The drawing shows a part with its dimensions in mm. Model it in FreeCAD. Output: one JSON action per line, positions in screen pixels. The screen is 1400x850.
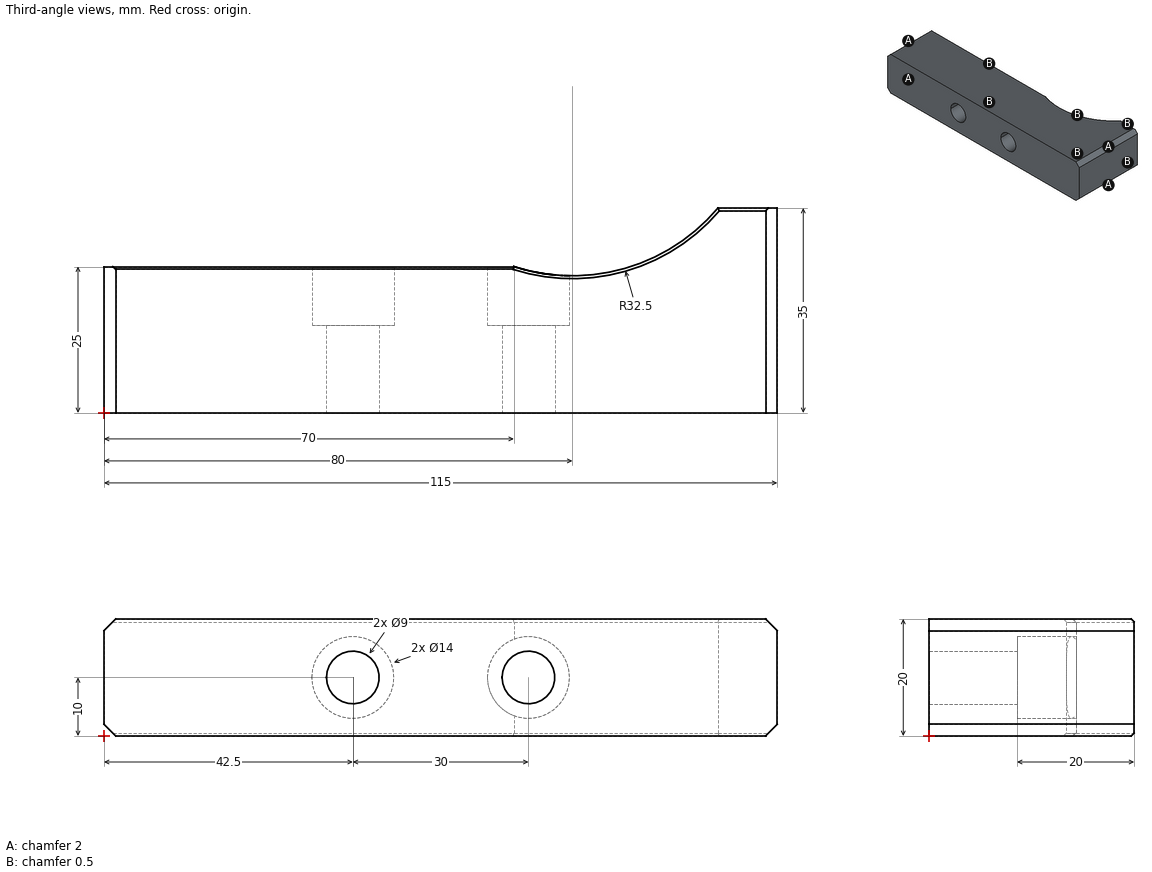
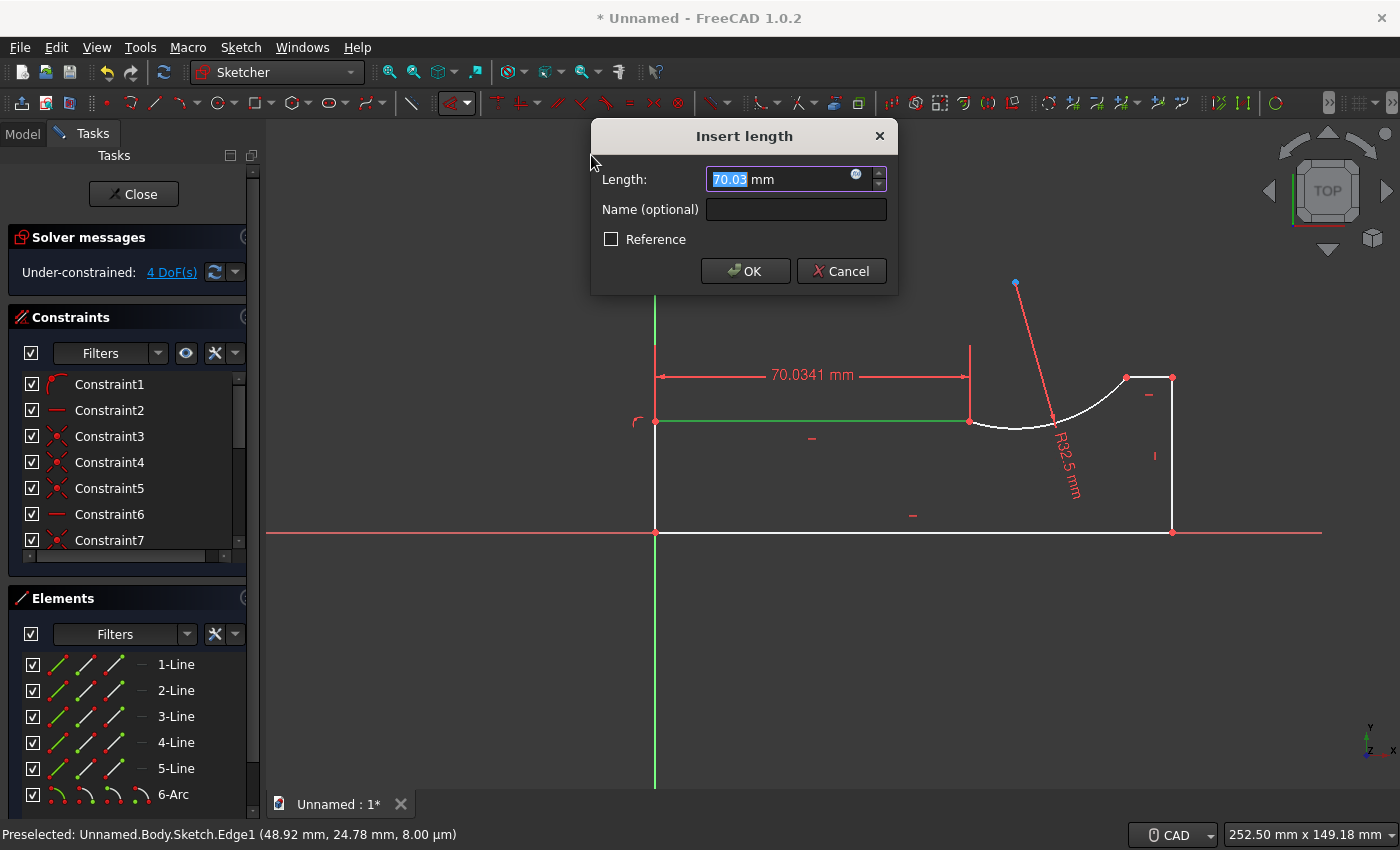
{"action": "type", "text": "70"}
{"action": "key", "text": "Return"}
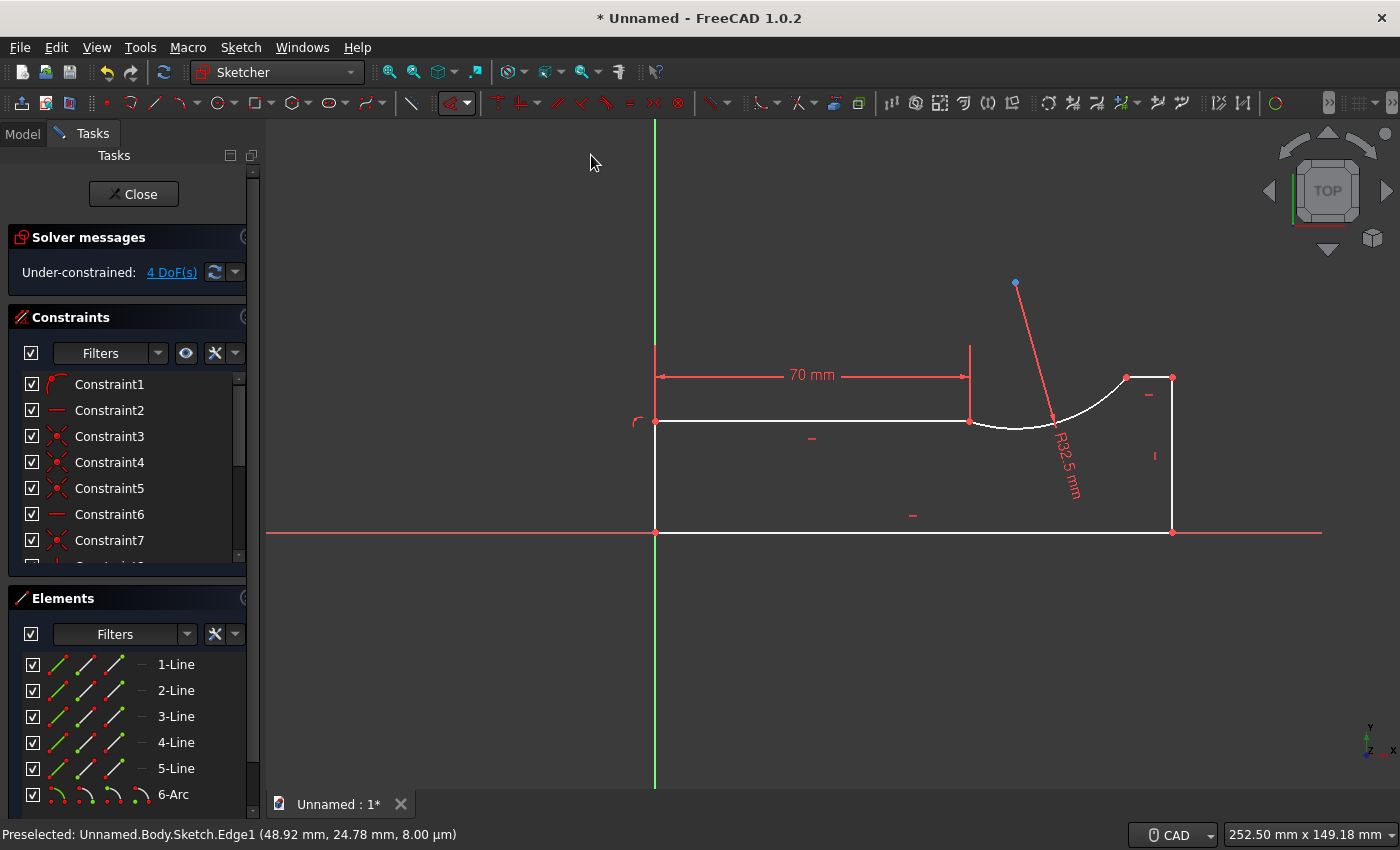
{"action": "left_click", "coordinate": [655, 455]}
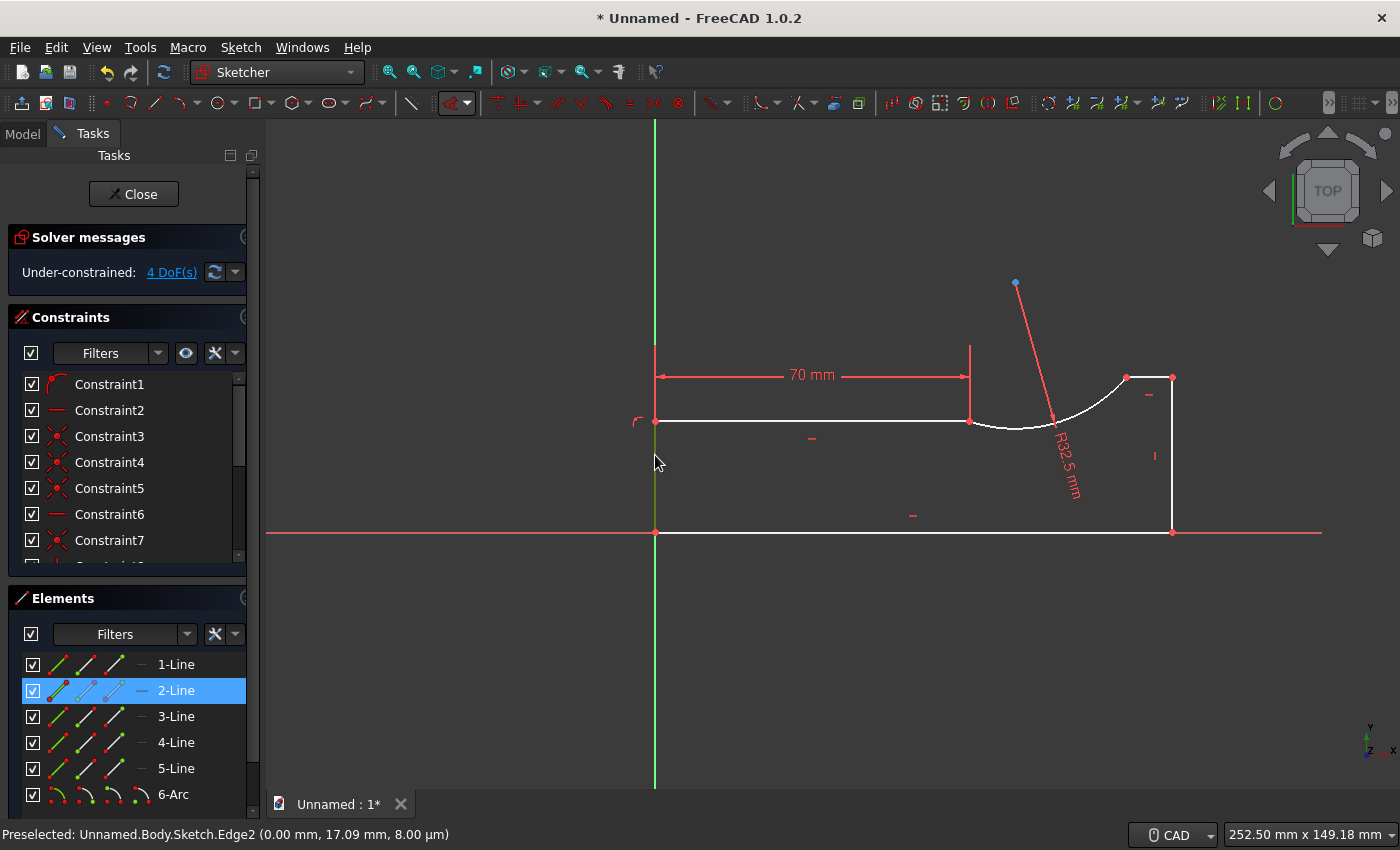
{"action": "key", "text": "i"}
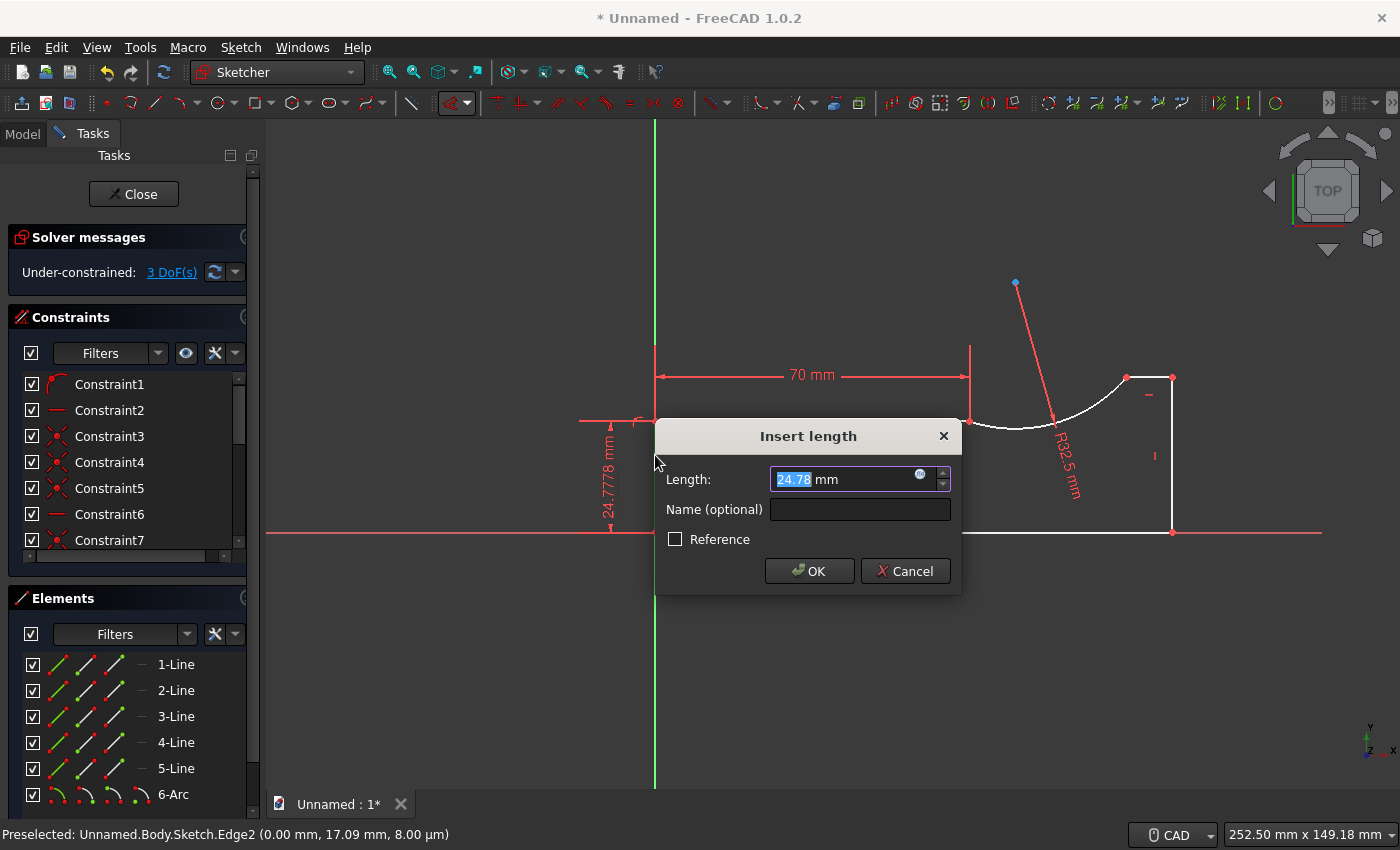
{"action": "type", "text": "25"}
{"action": "key", "text": "Return"}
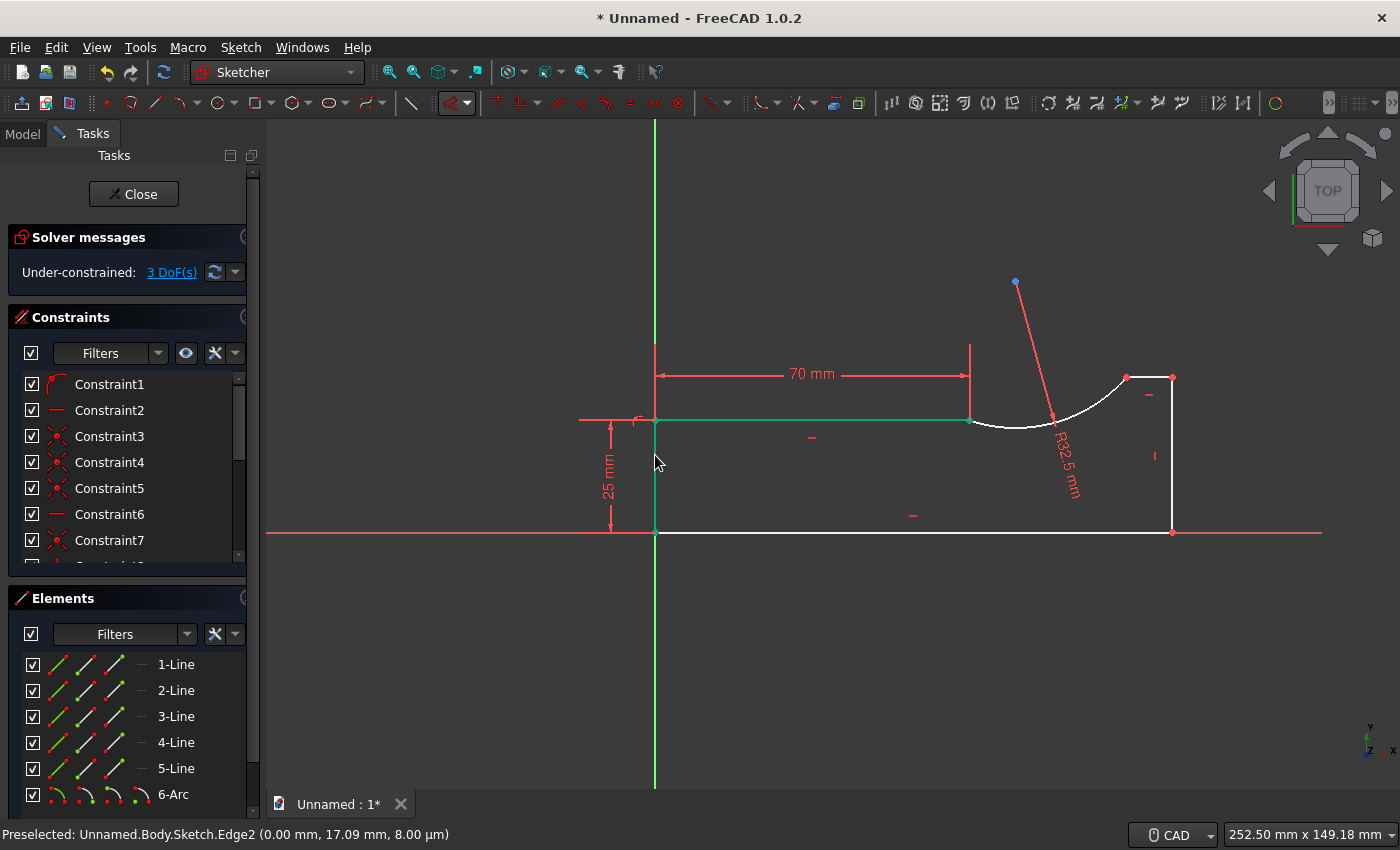
{"action": "left_click", "coordinate": [1172, 486]}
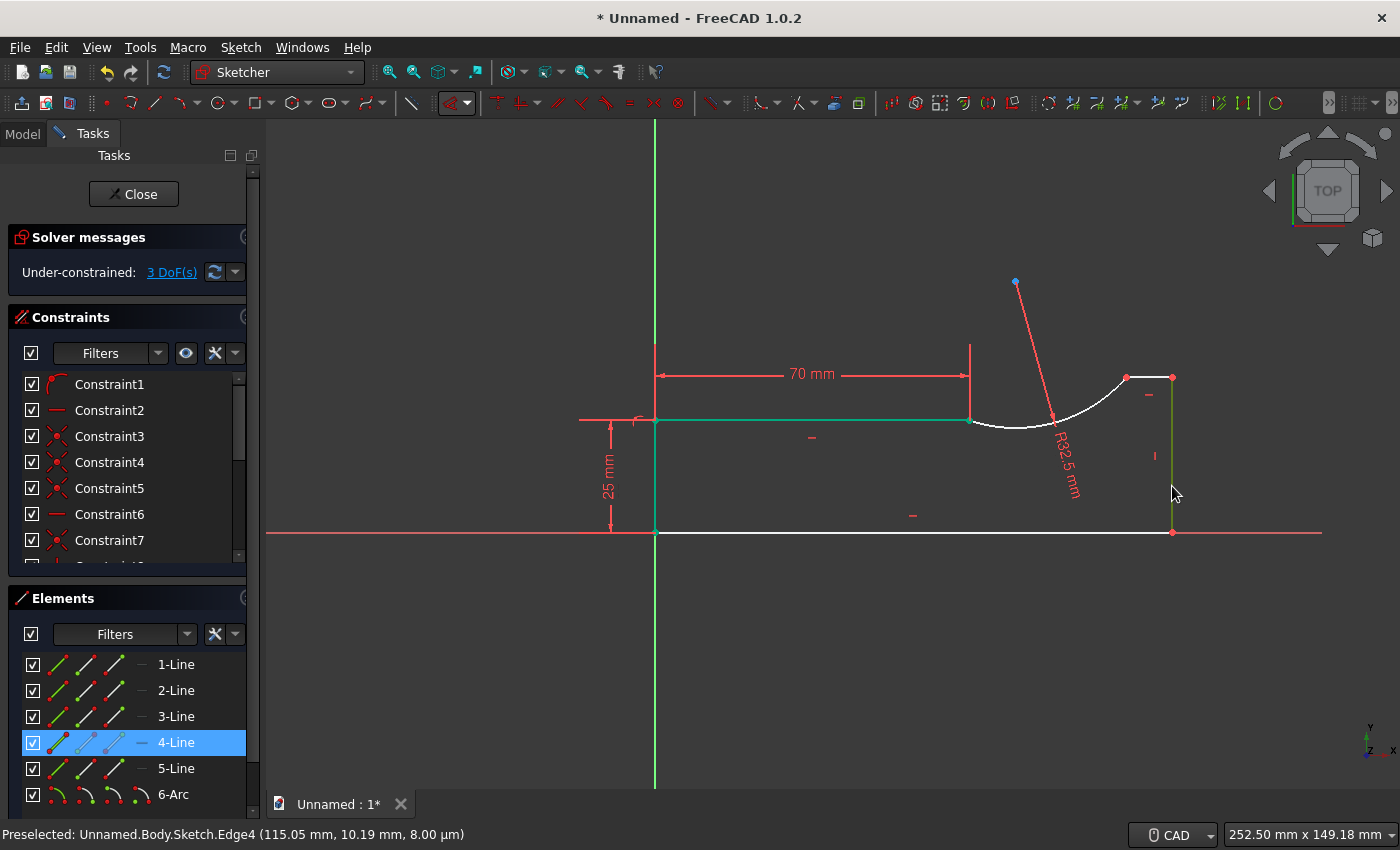
{"action": "key", "text": "i"}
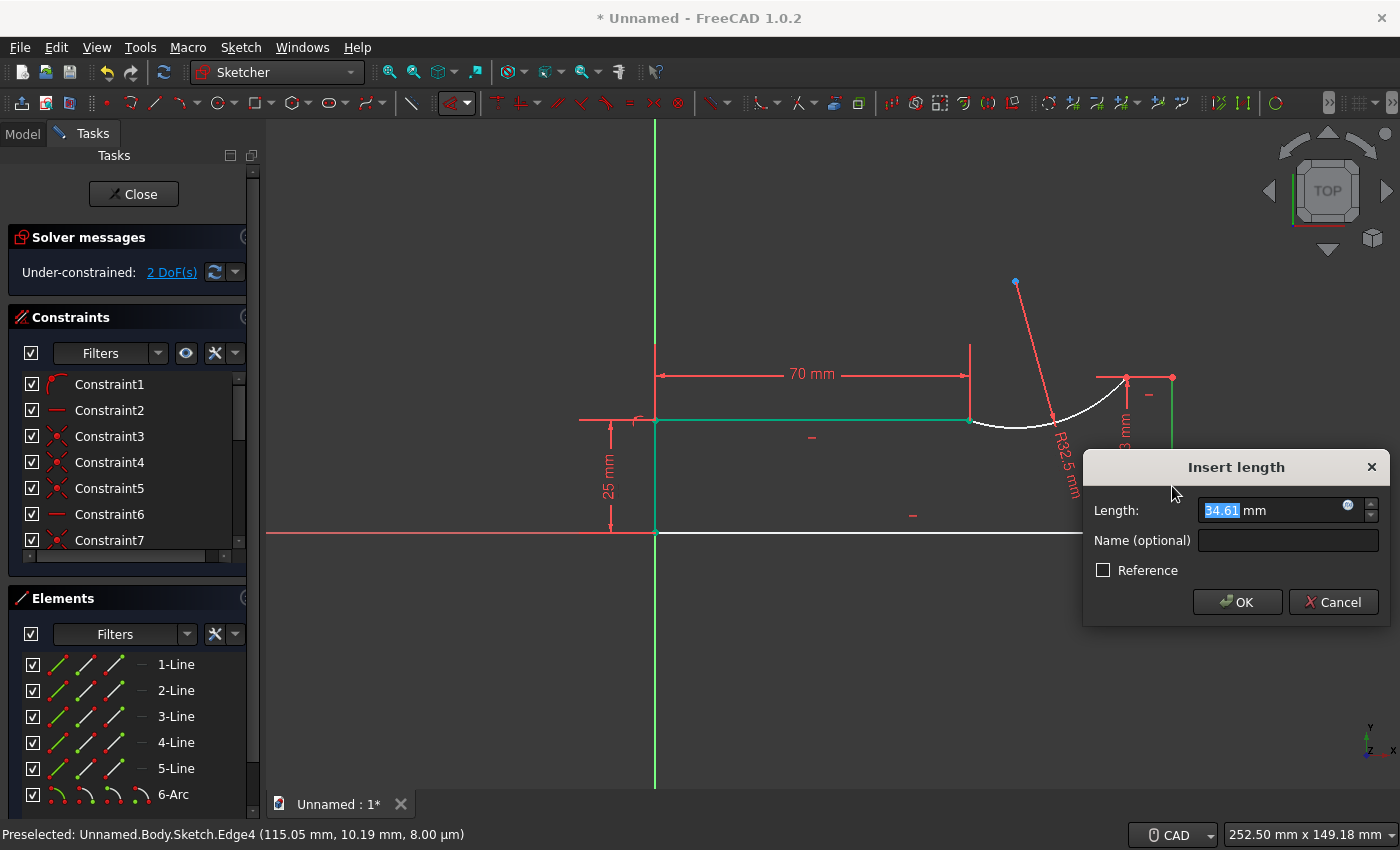
{"action": "type", "text": "35"}
{"action": "key", "text": "Return"}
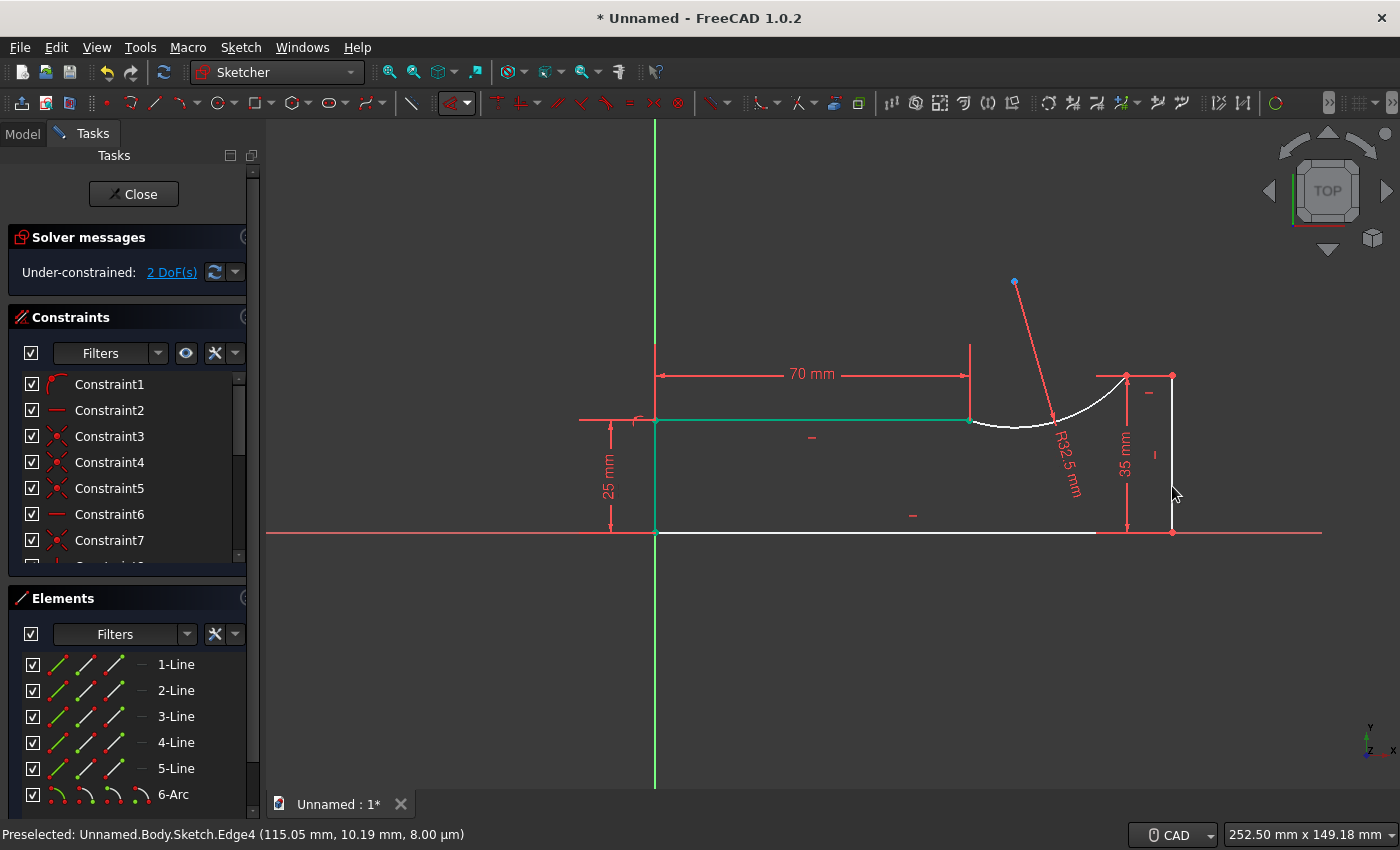
{"action": "left_click", "coordinate": [810, 533]}